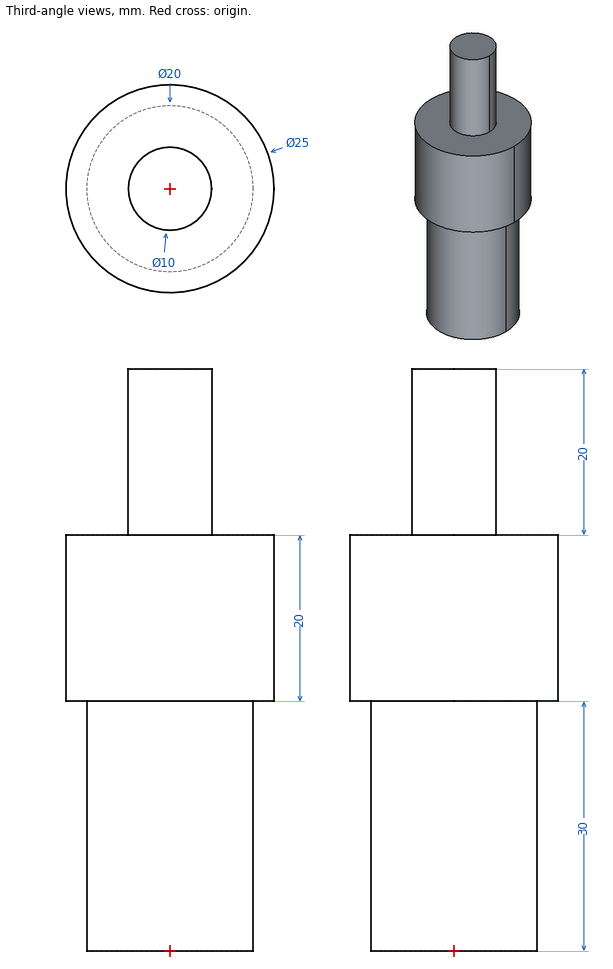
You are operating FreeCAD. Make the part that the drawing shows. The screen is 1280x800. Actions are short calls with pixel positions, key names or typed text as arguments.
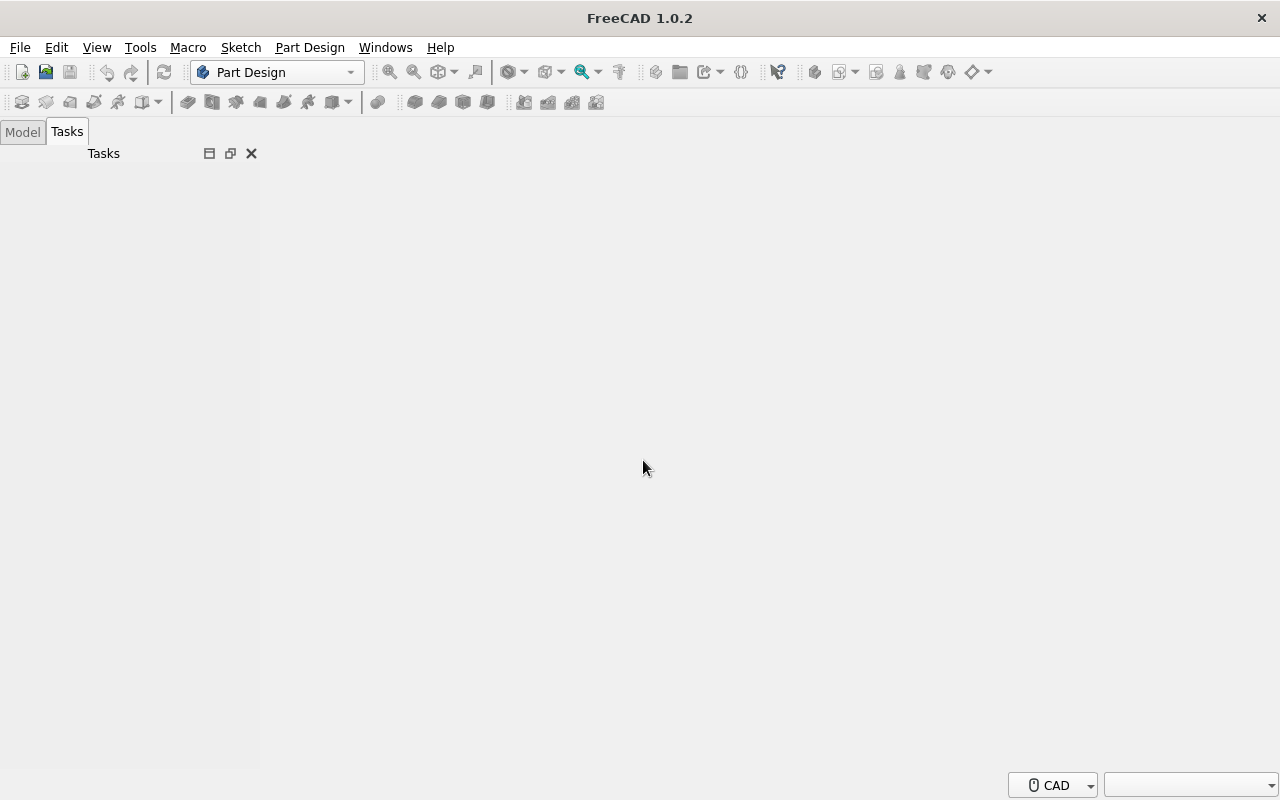
key(ctrl+n)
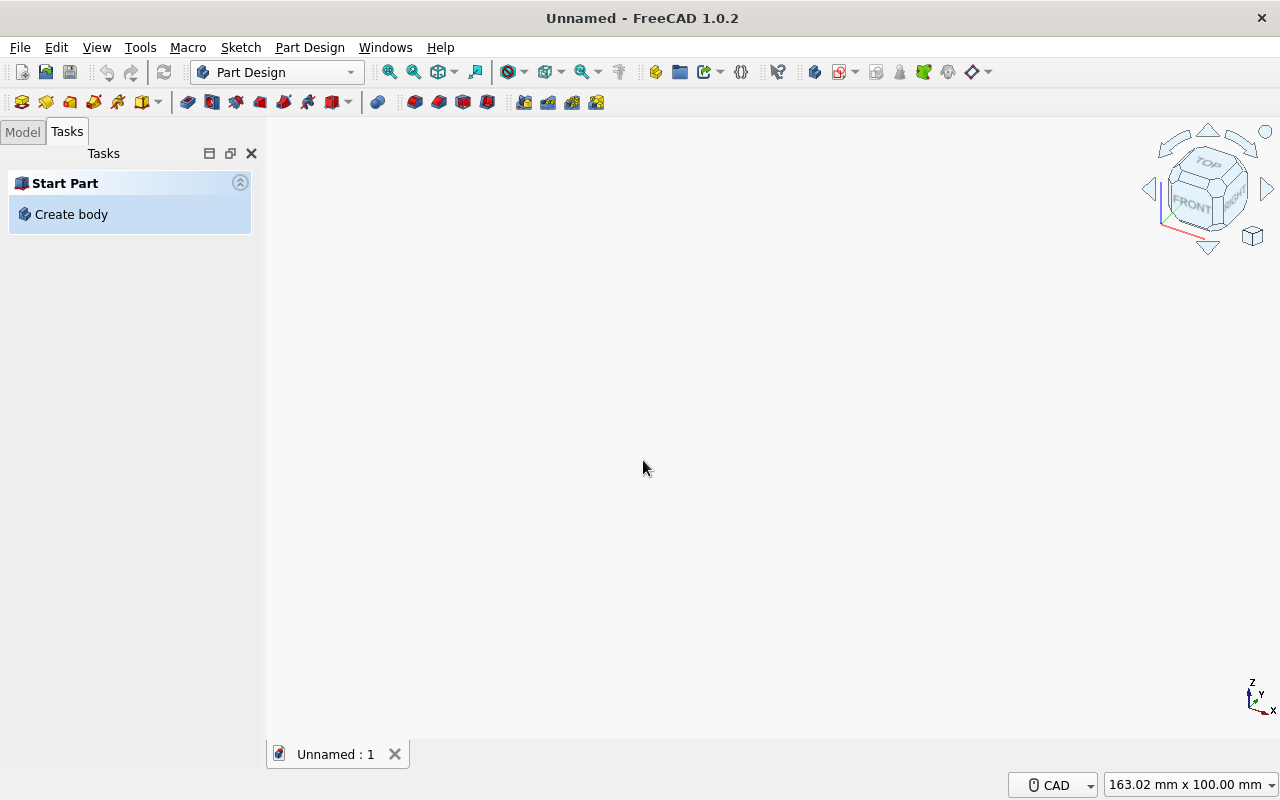
click(840, 72)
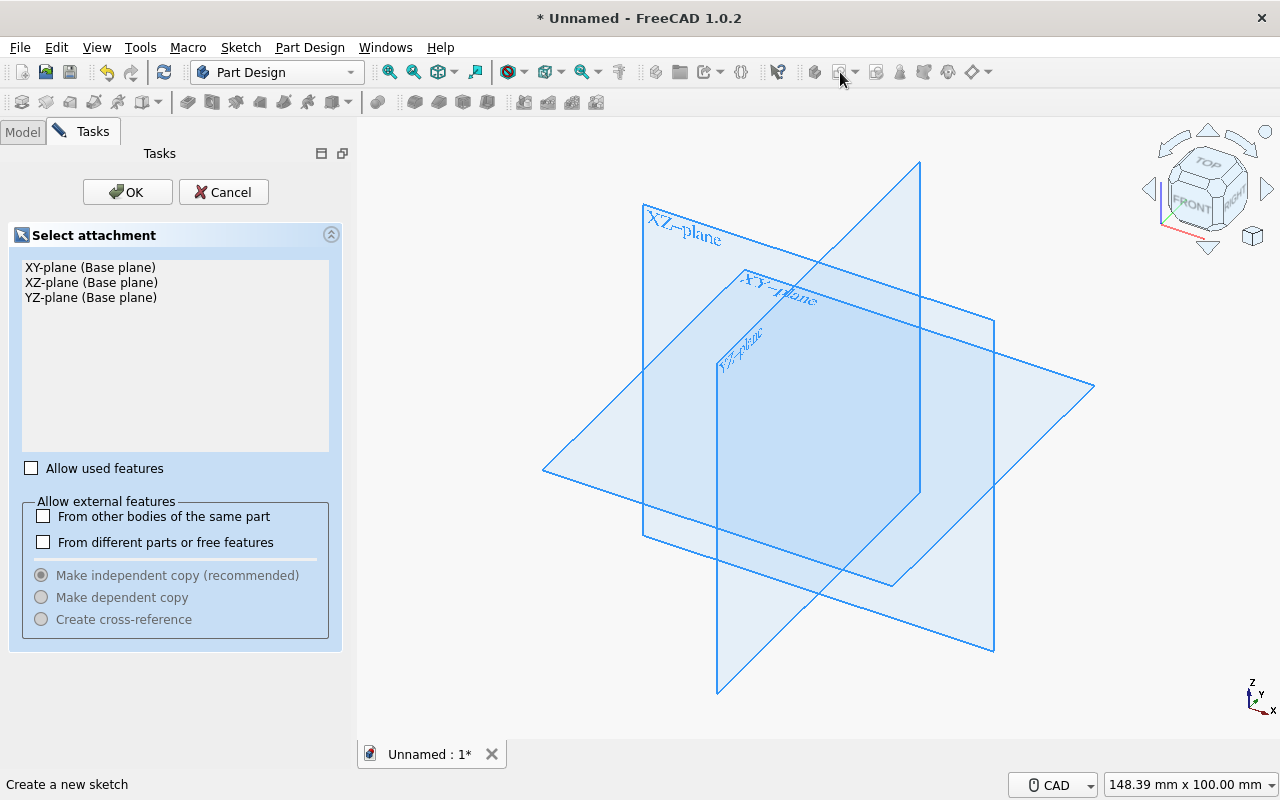
click(82, 268)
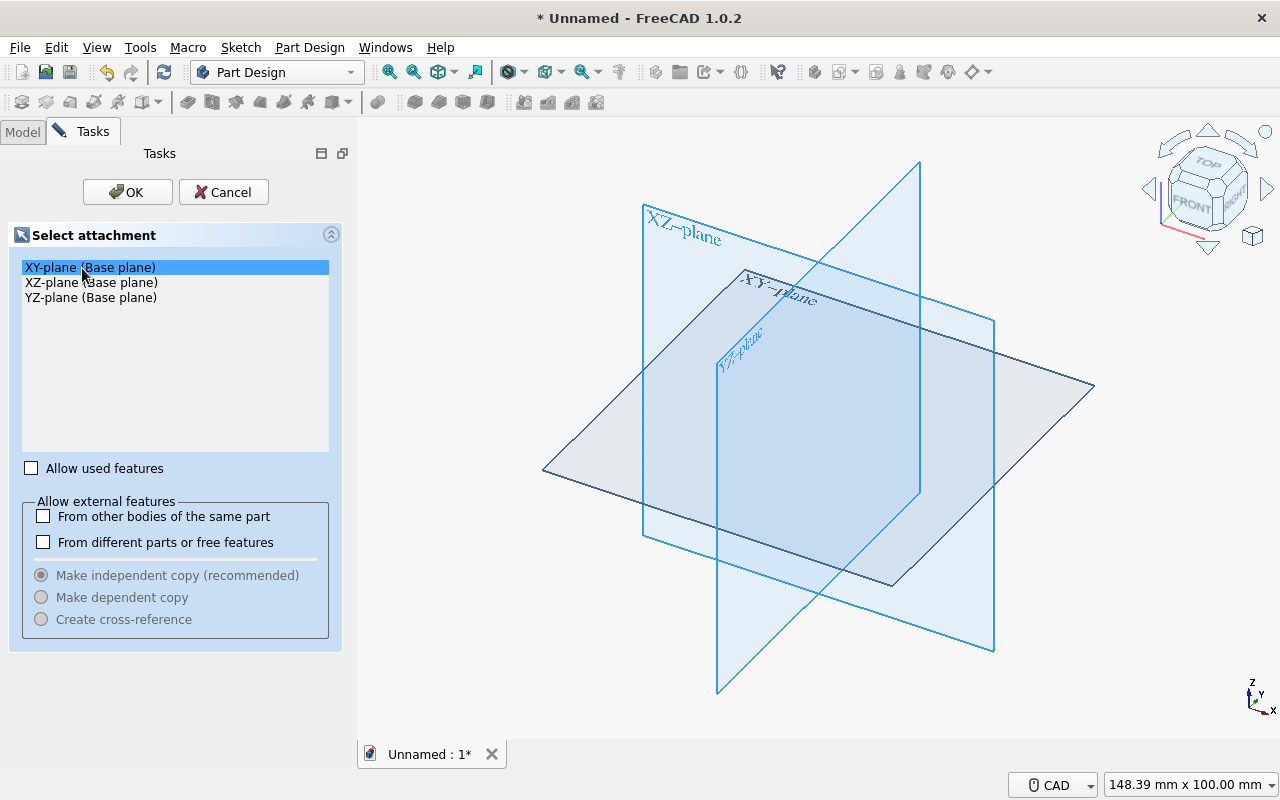
click(128, 192)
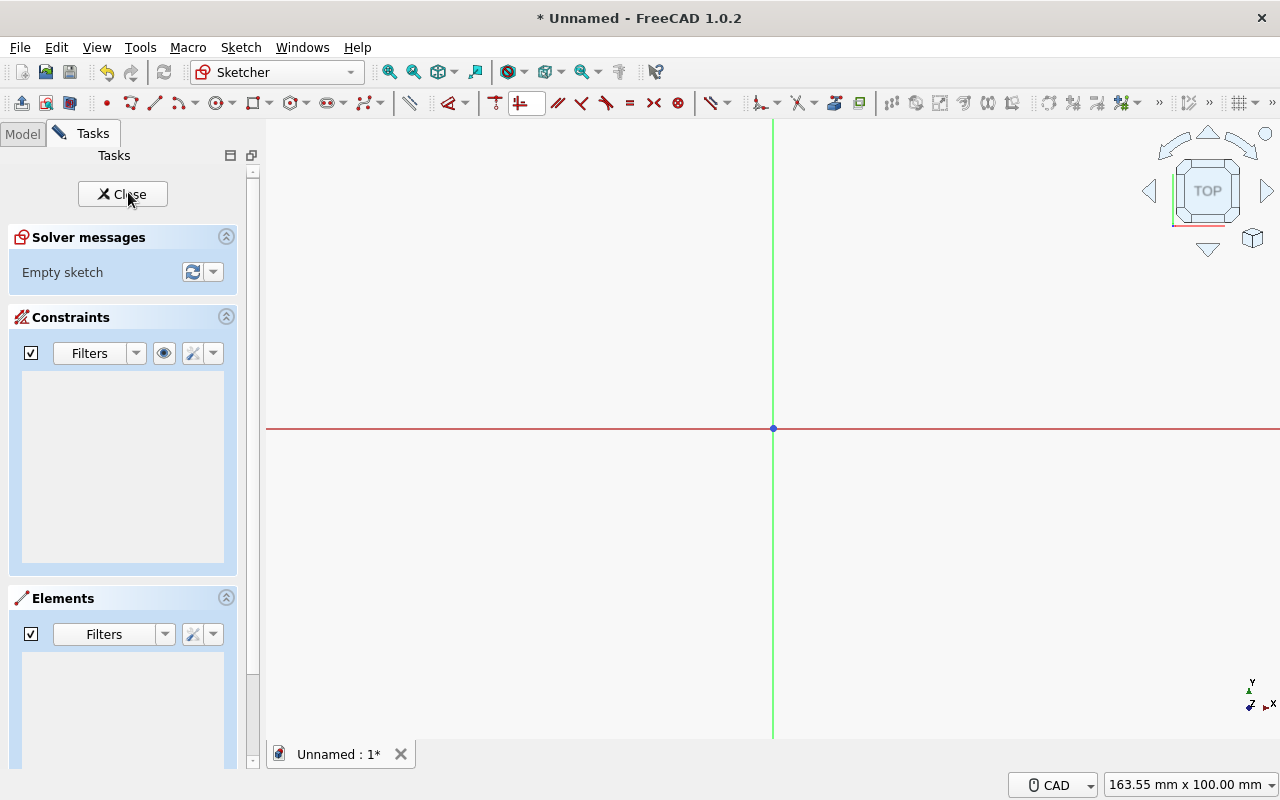
scroll(803, 429, up, 6)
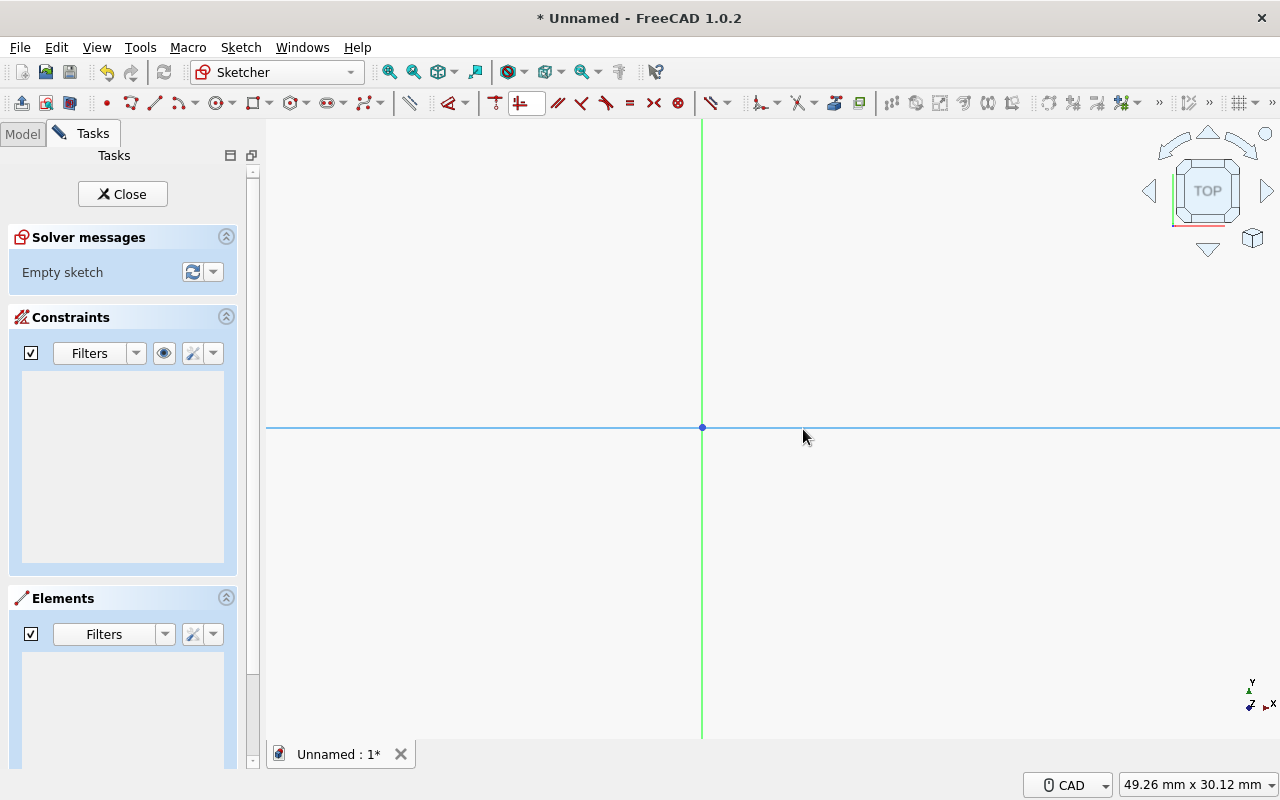
click(216, 104)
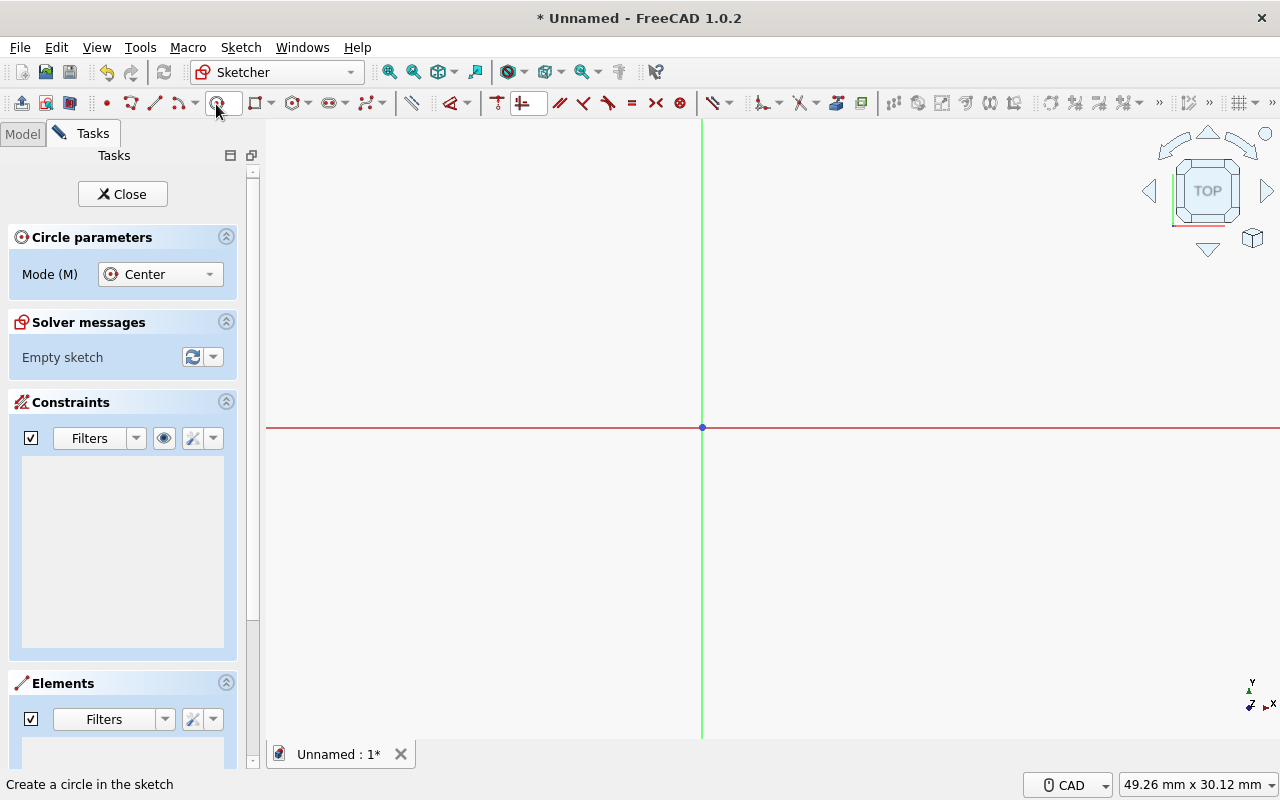
click(702, 428)
click(848, 282)
key(Escape)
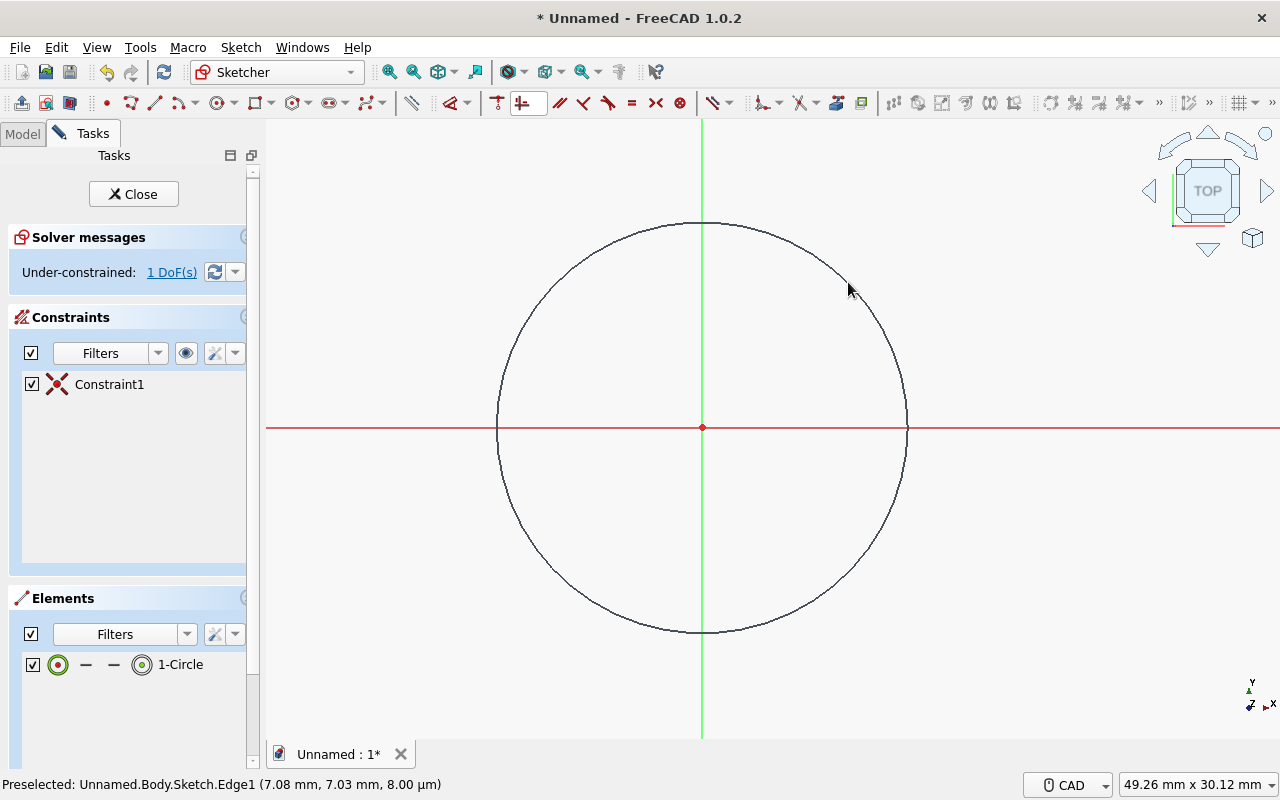
key(d)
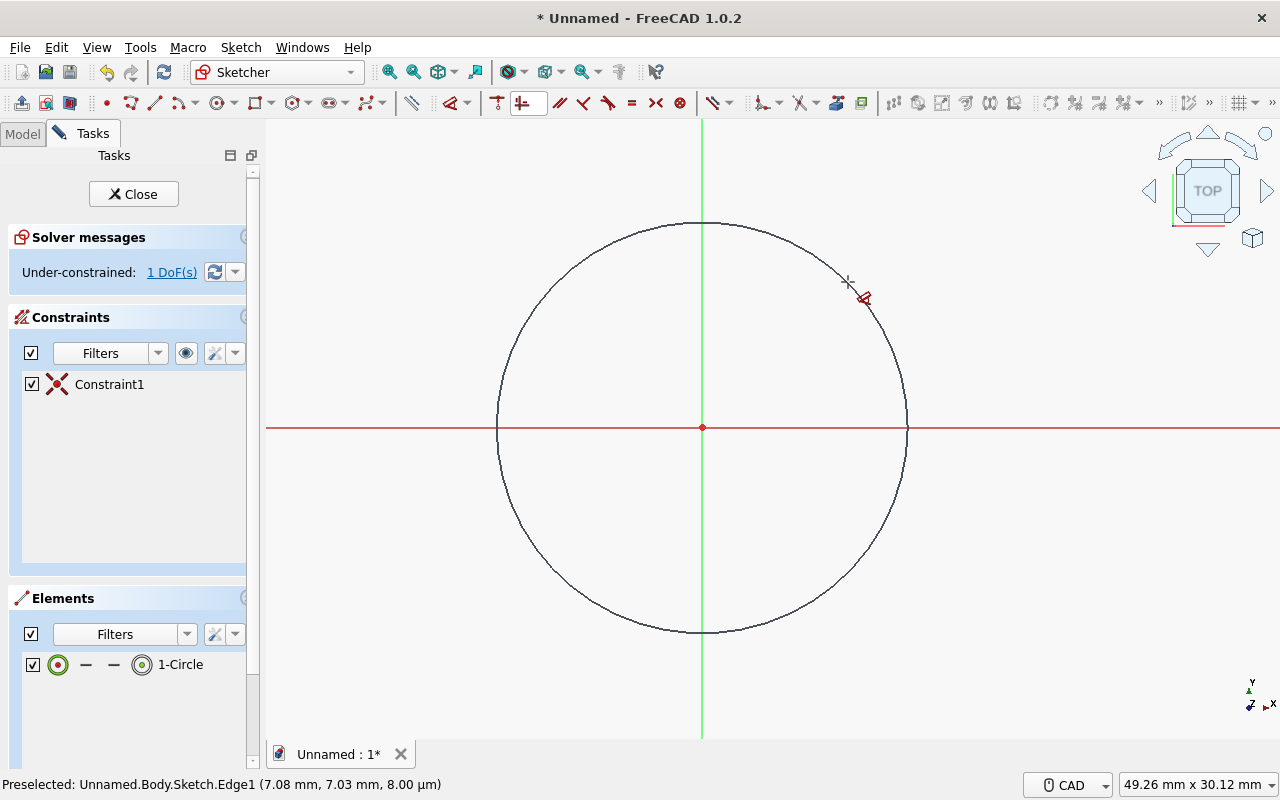
click(847, 282)
click(870, 259)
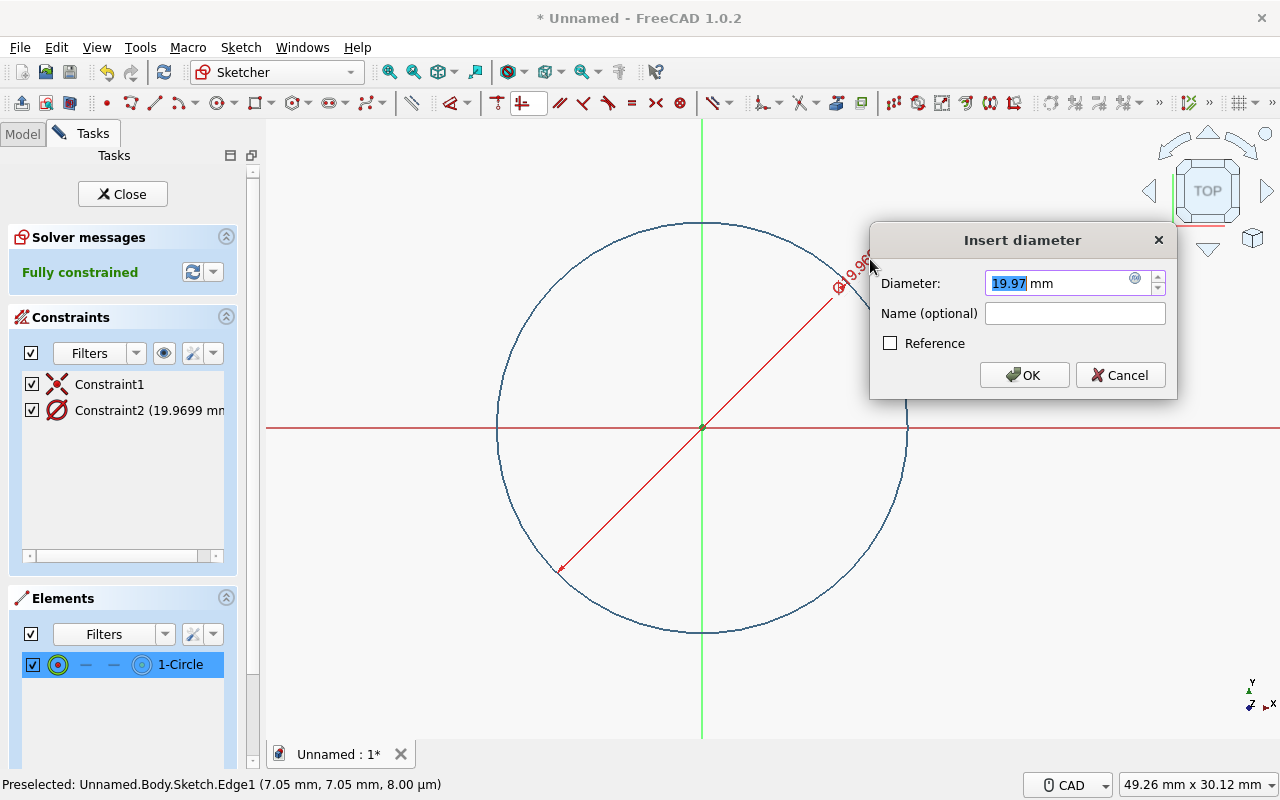
text(20)
key(Return)
key(Escape)